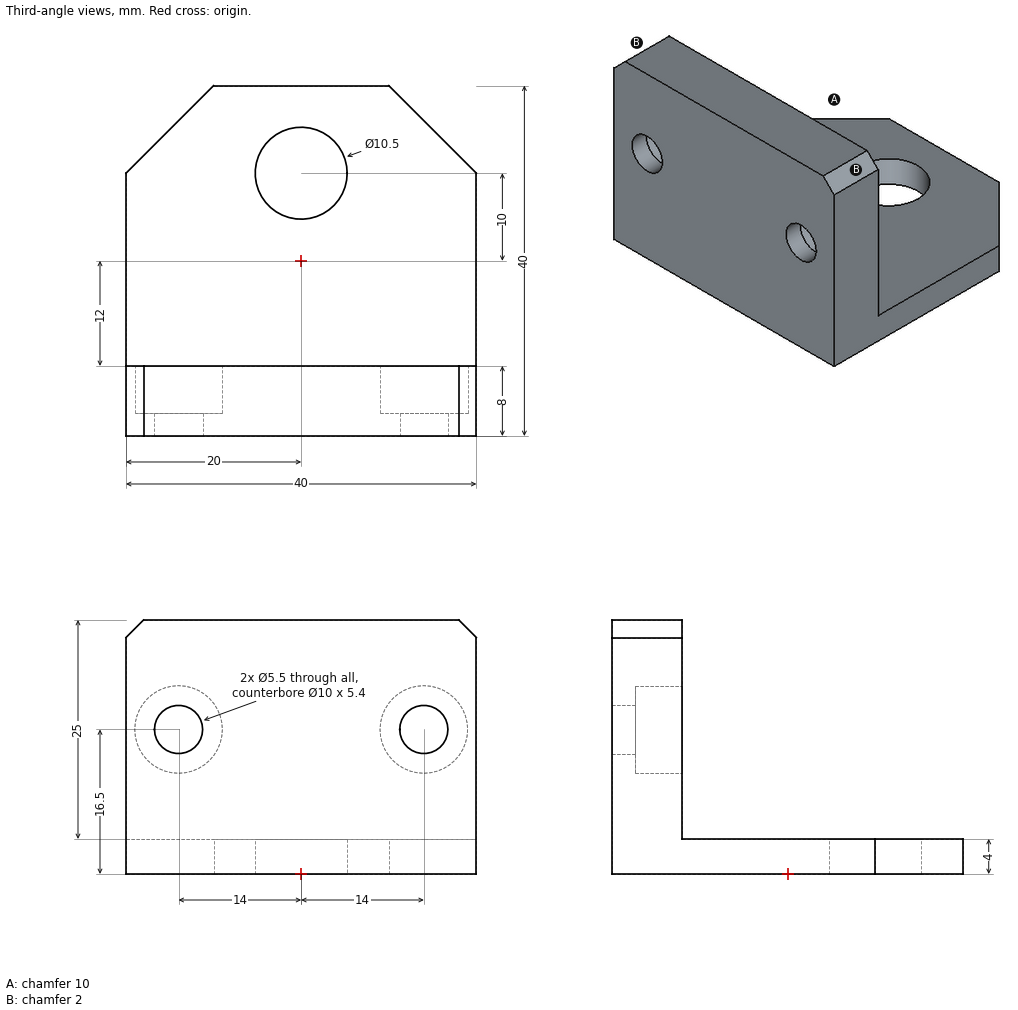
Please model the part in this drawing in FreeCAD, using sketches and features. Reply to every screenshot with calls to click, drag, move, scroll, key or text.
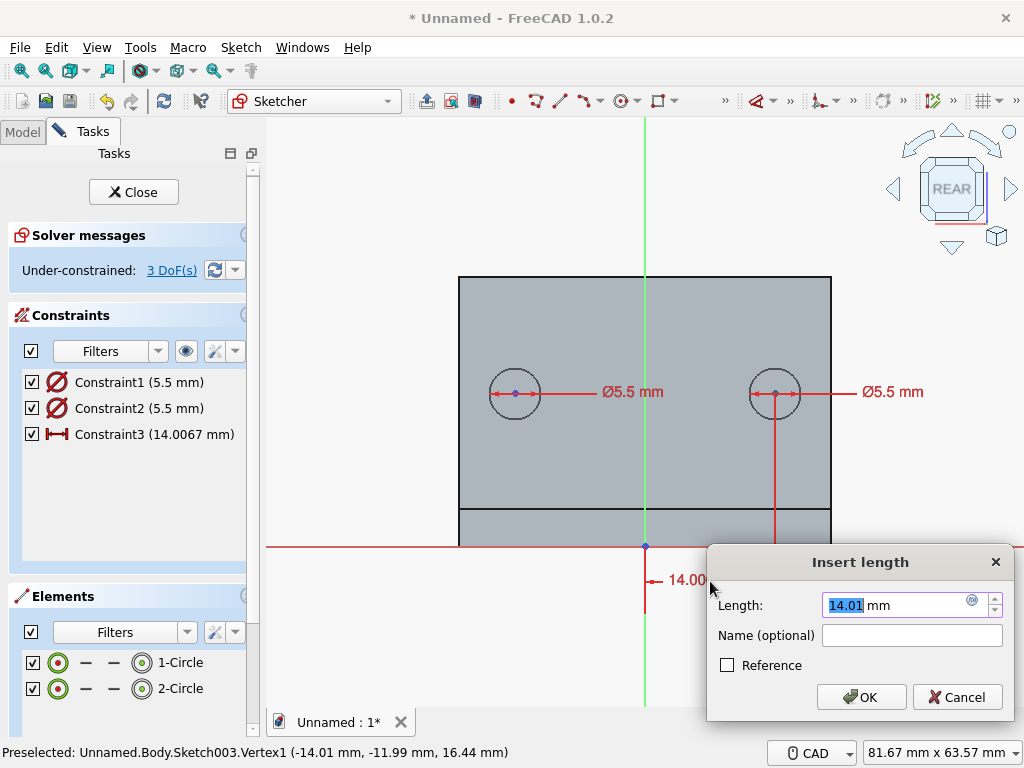
text(14)
key(Return)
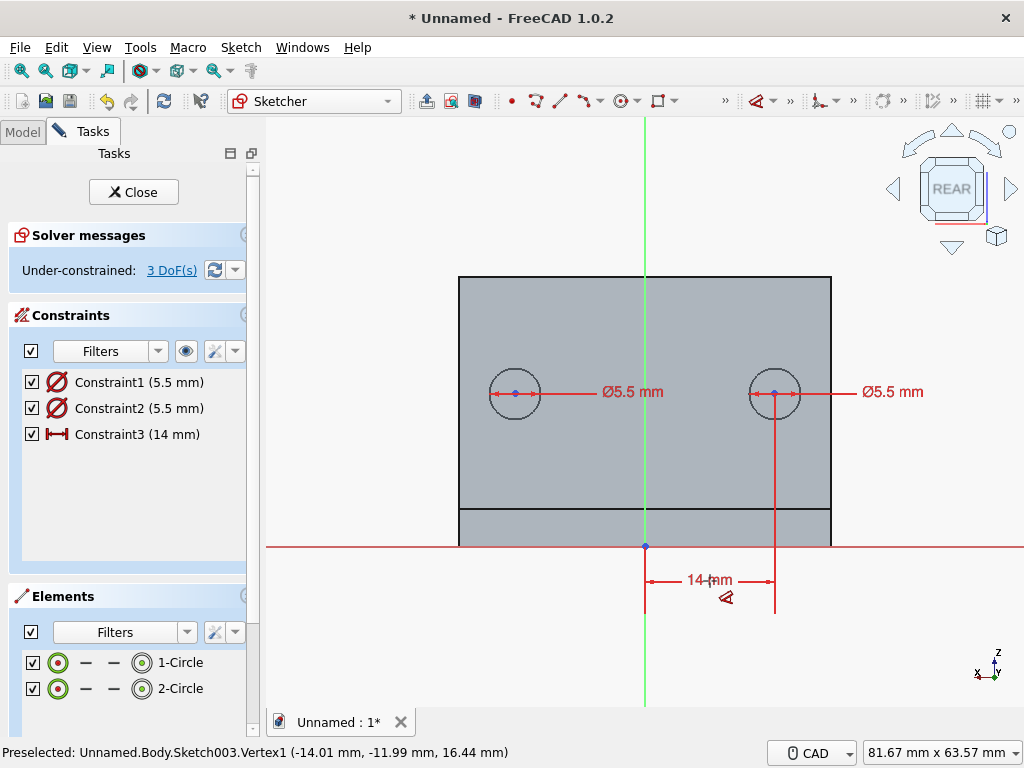
click(515, 394)
click(580, 581)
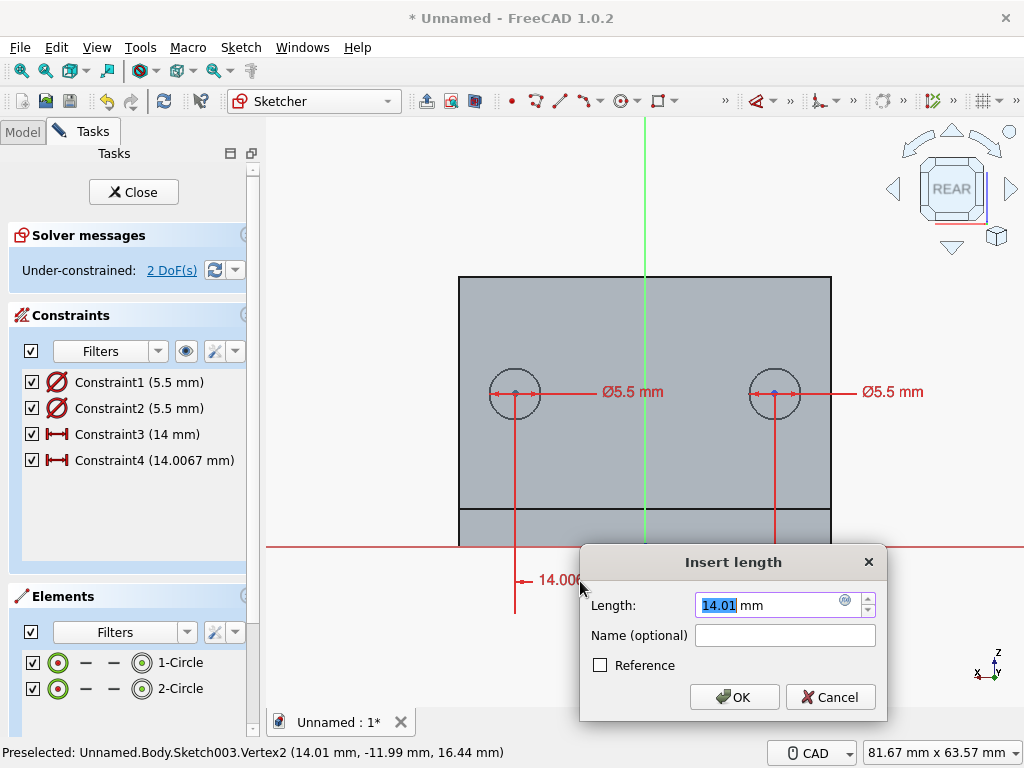
text(14)
key(Return)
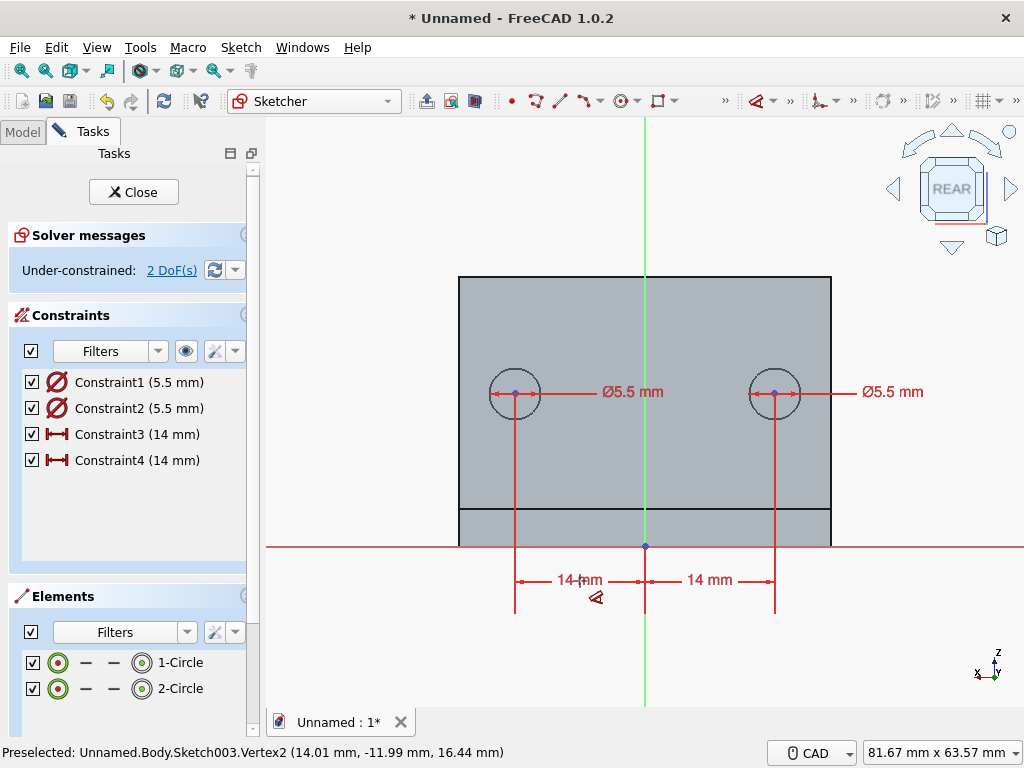
click(775, 394)
click(809, 470)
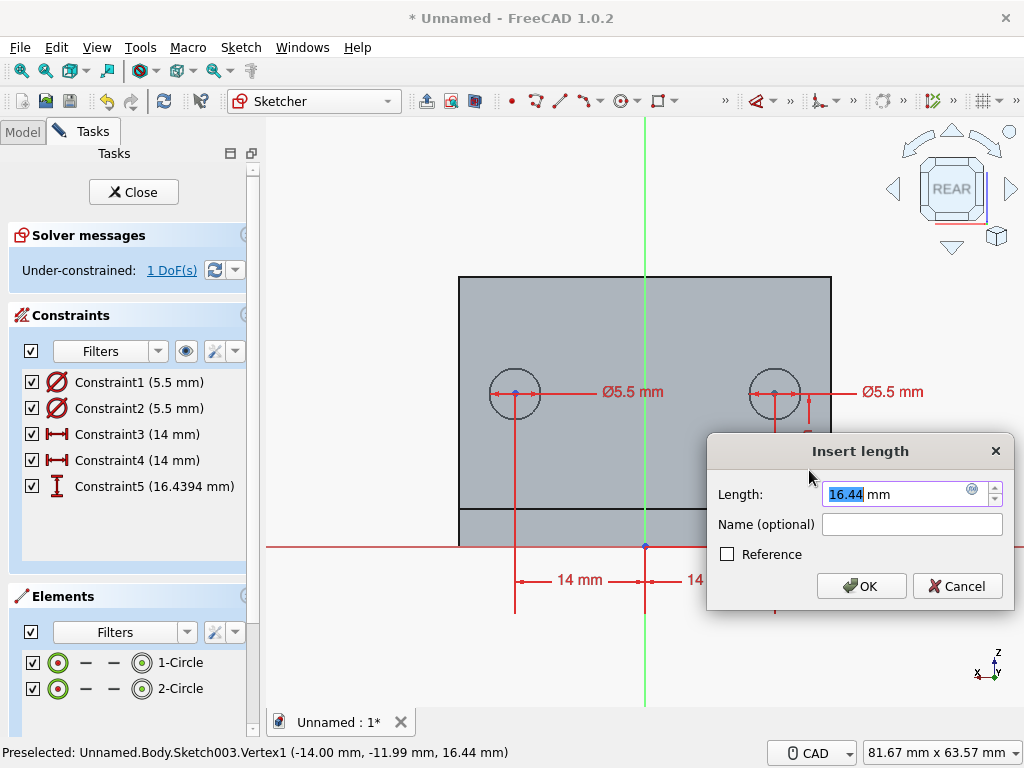
text(16.5)
key(Return)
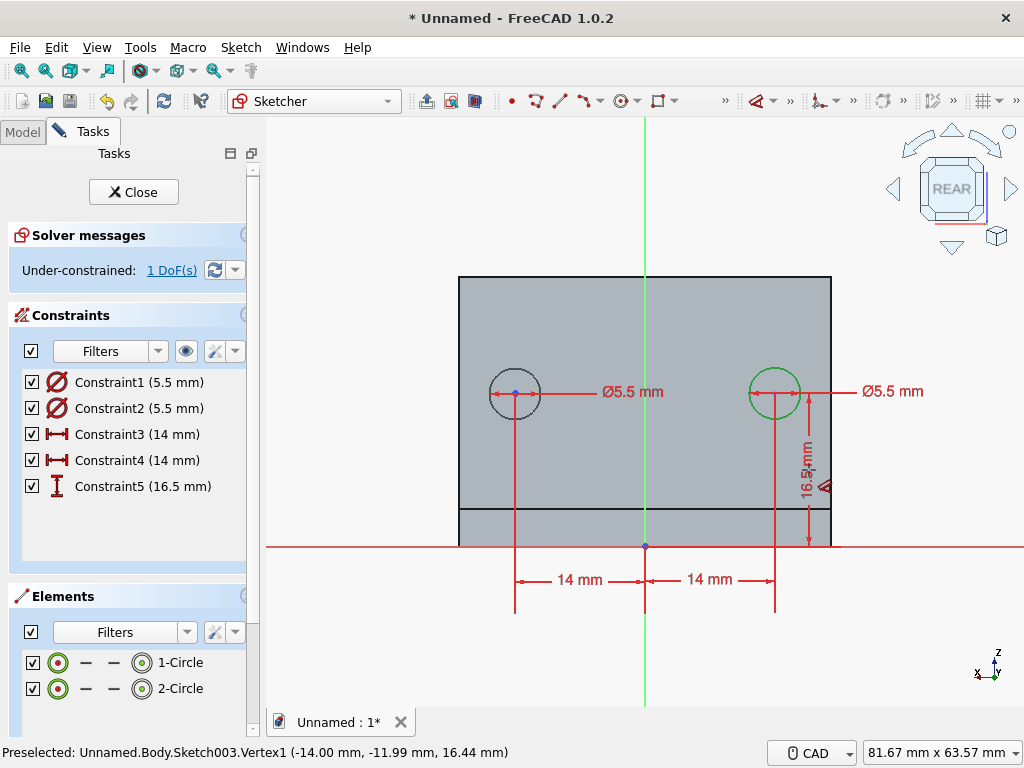
click(515, 394)
click(481, 470)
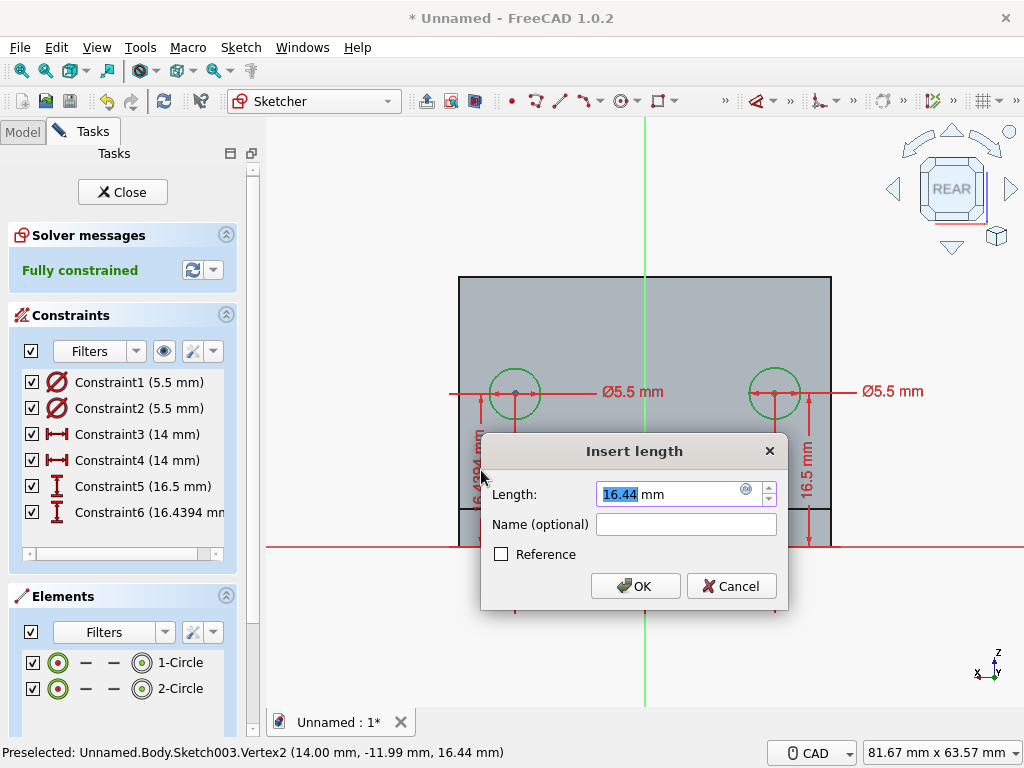
text(16.5)
key(Return)
key(Escape)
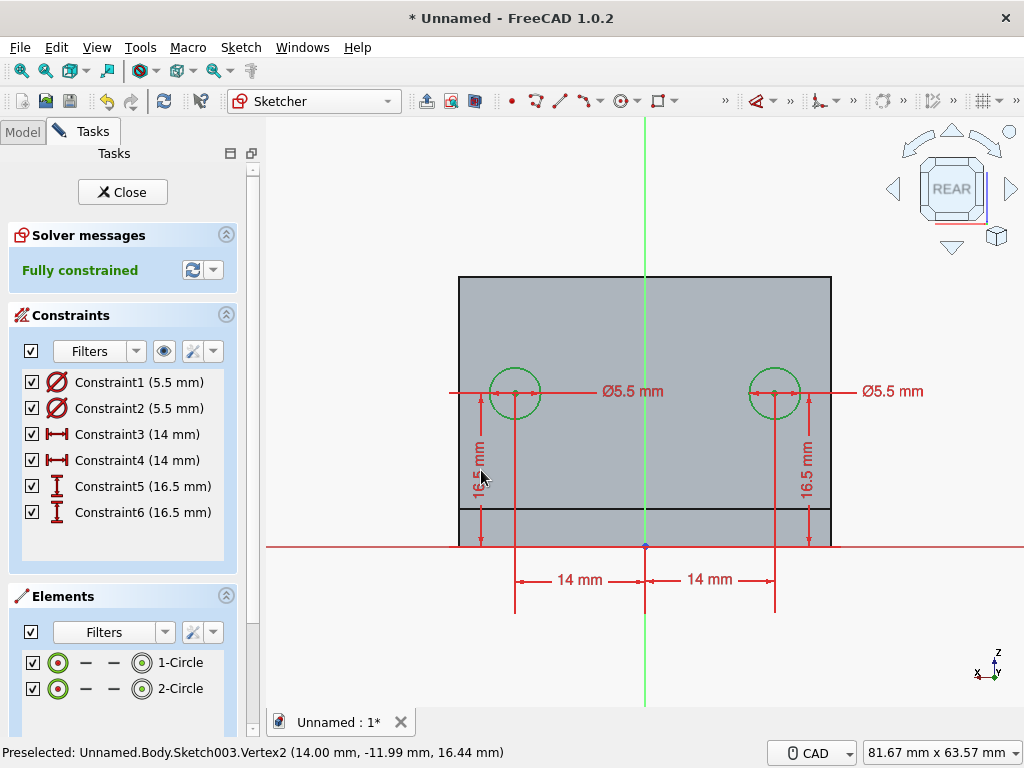
click(123, 192)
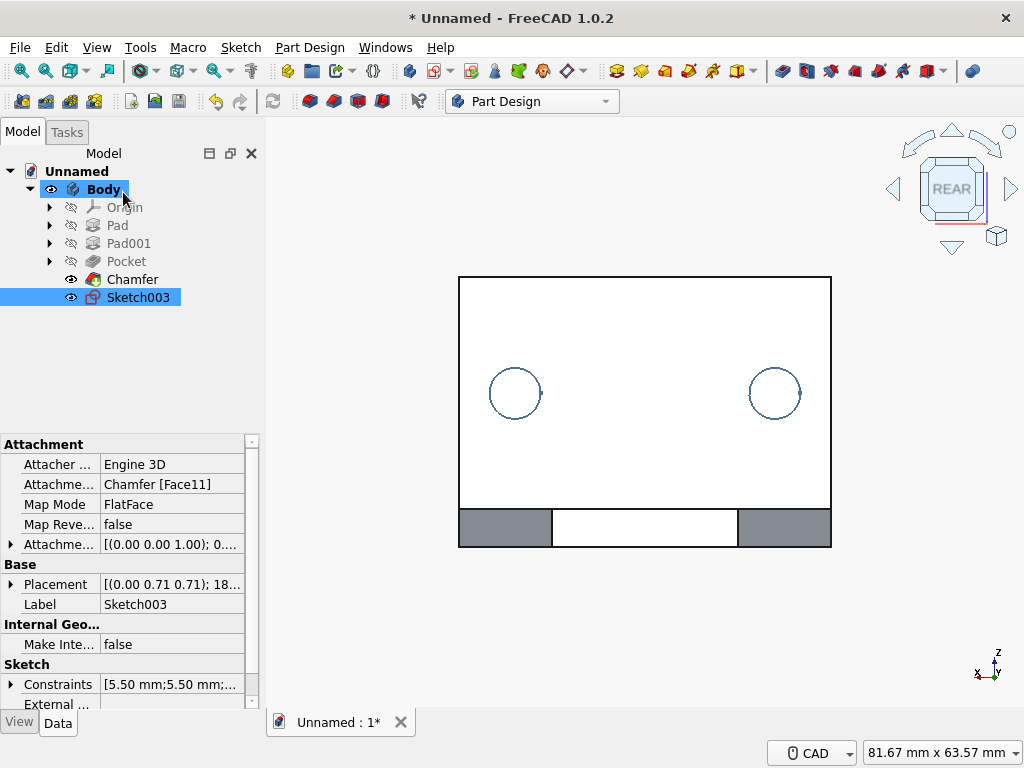
click(808, 72)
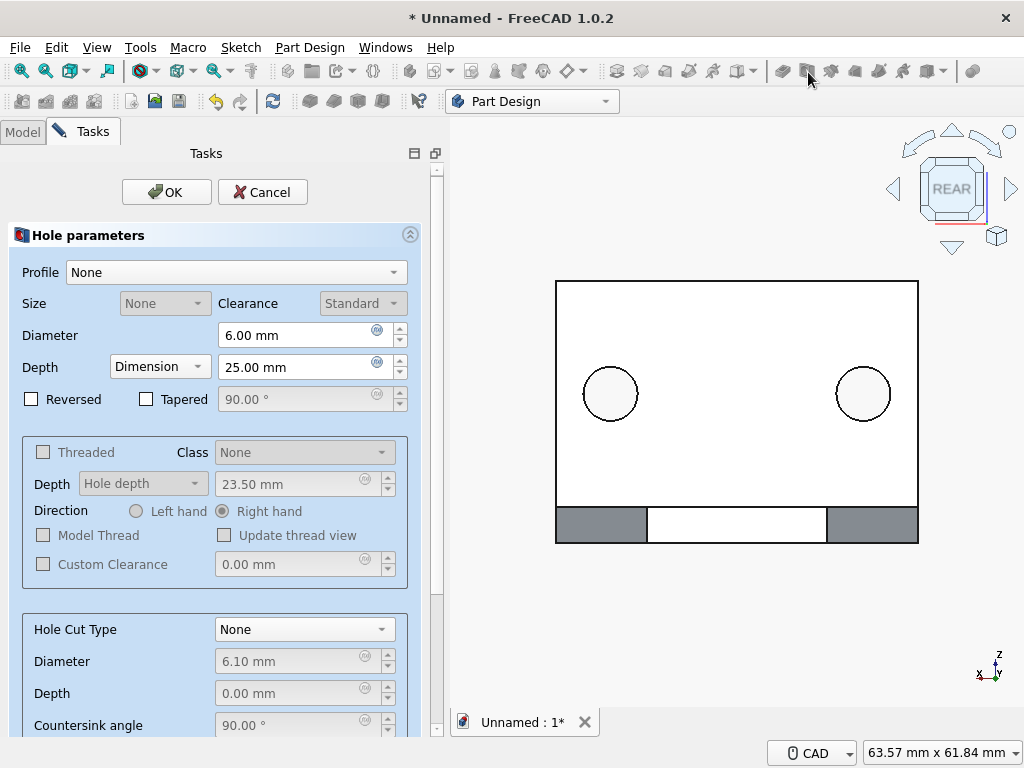
triple_click(305, 335)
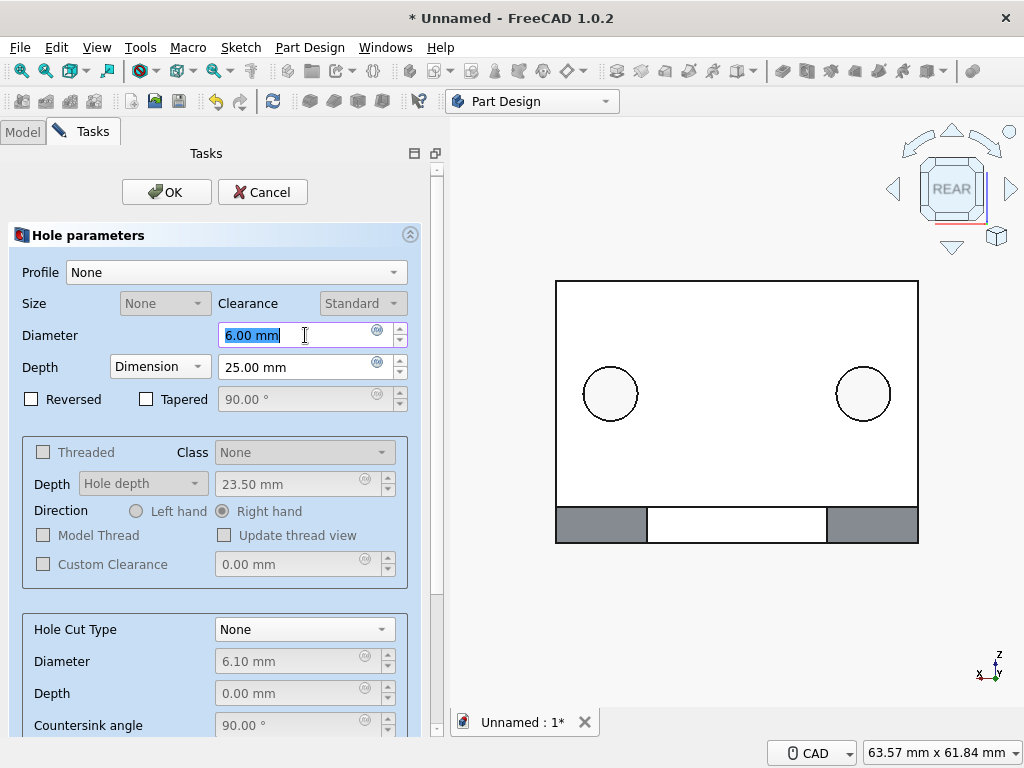
text(5.5)
key(Tab)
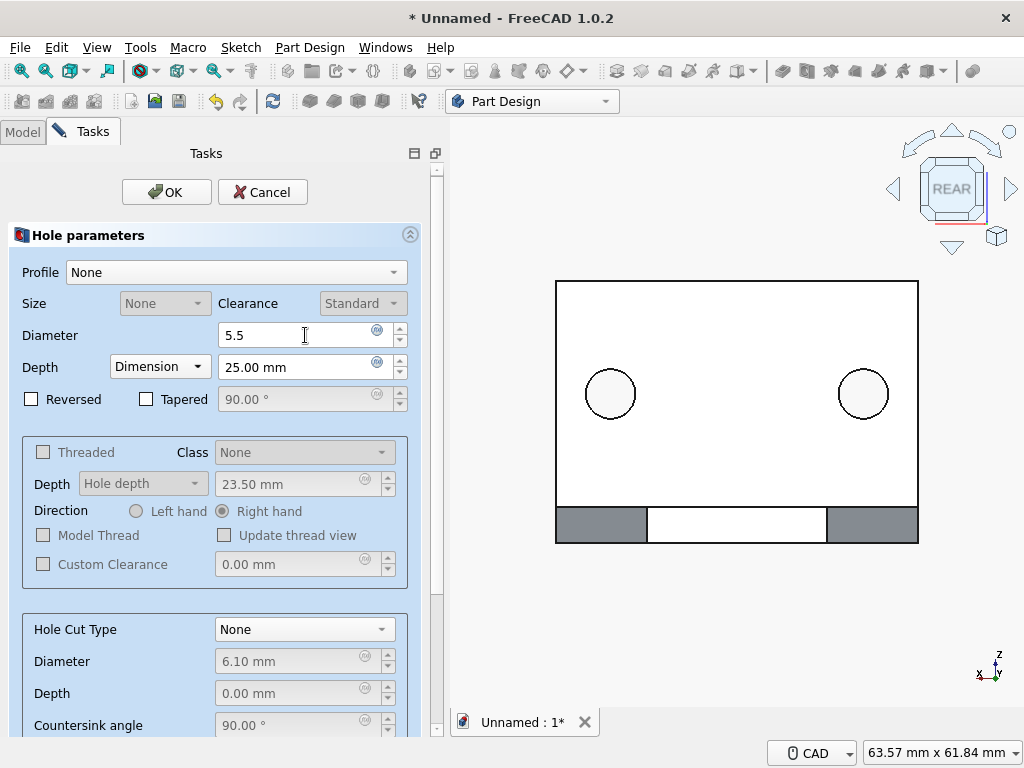
click(161, 366)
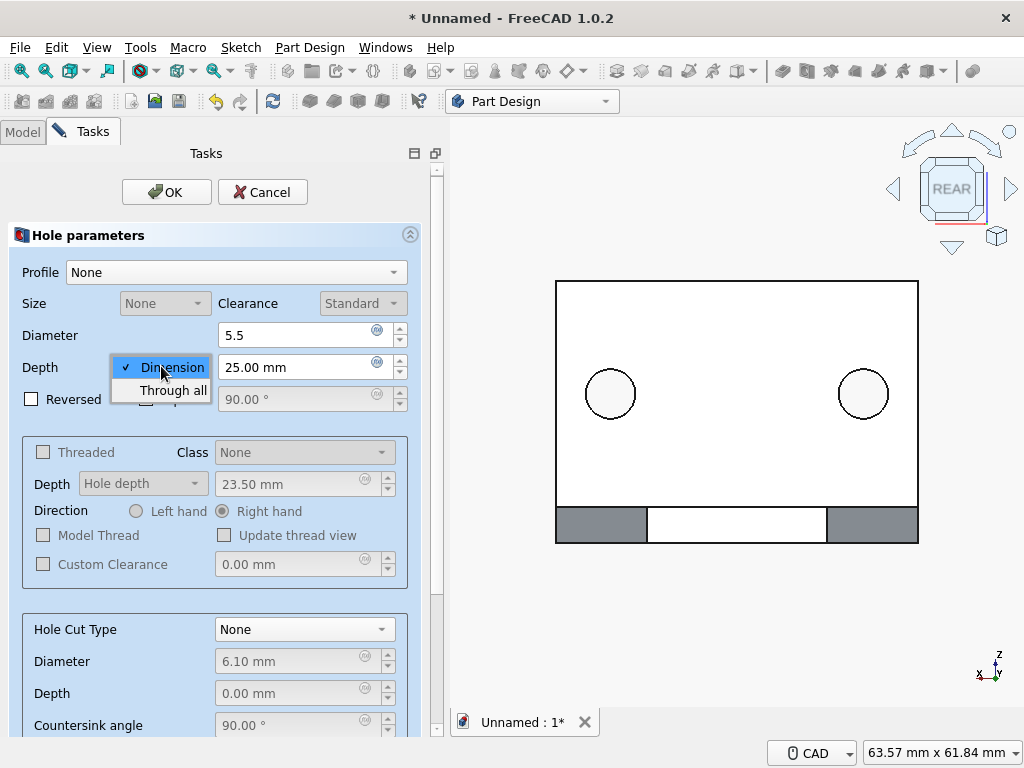
click(160, 390)